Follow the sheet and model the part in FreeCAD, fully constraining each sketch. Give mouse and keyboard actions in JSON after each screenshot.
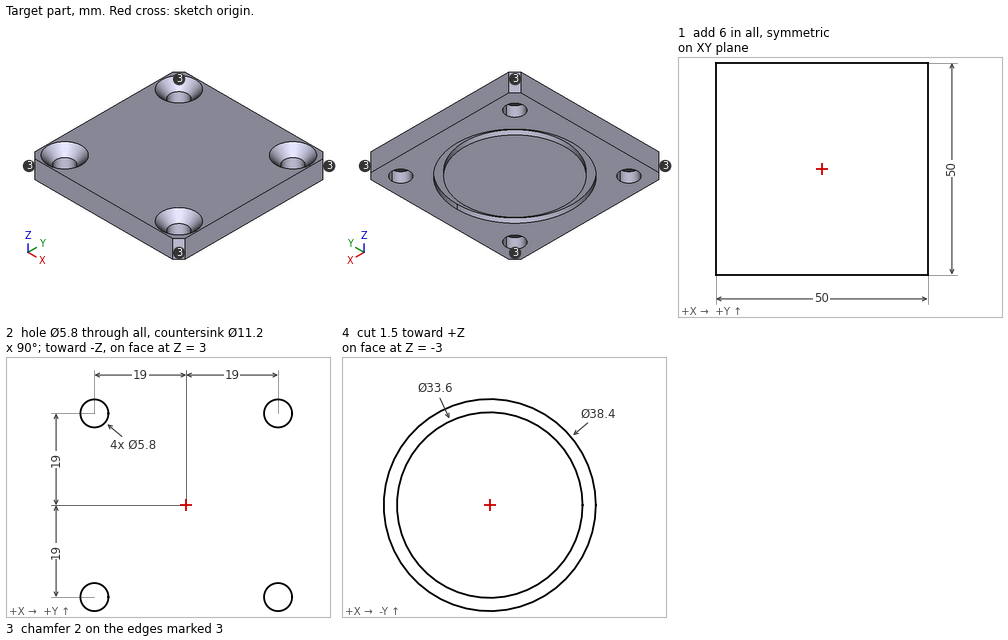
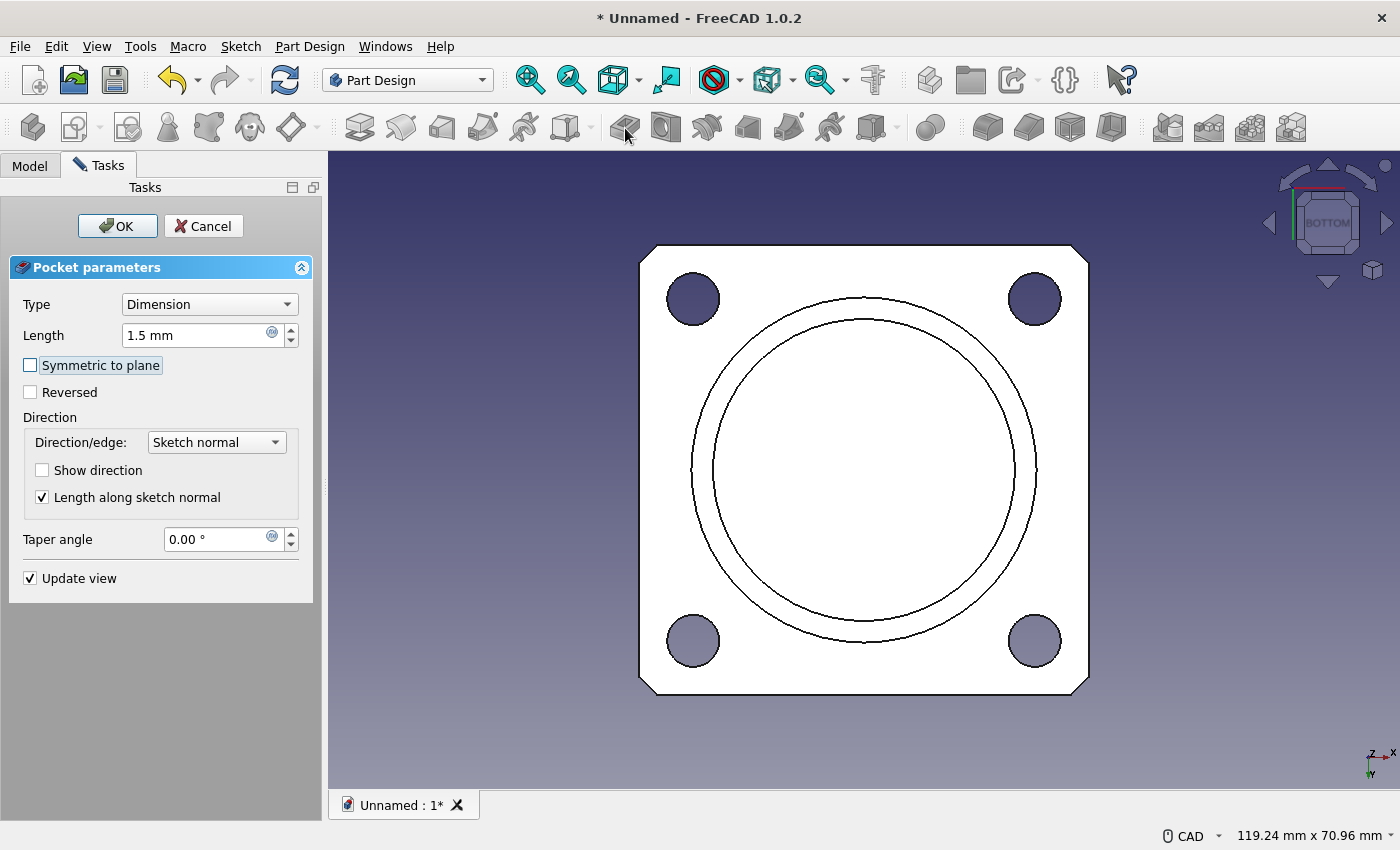
{"action": "left_click", "coordinate": [118, 226]}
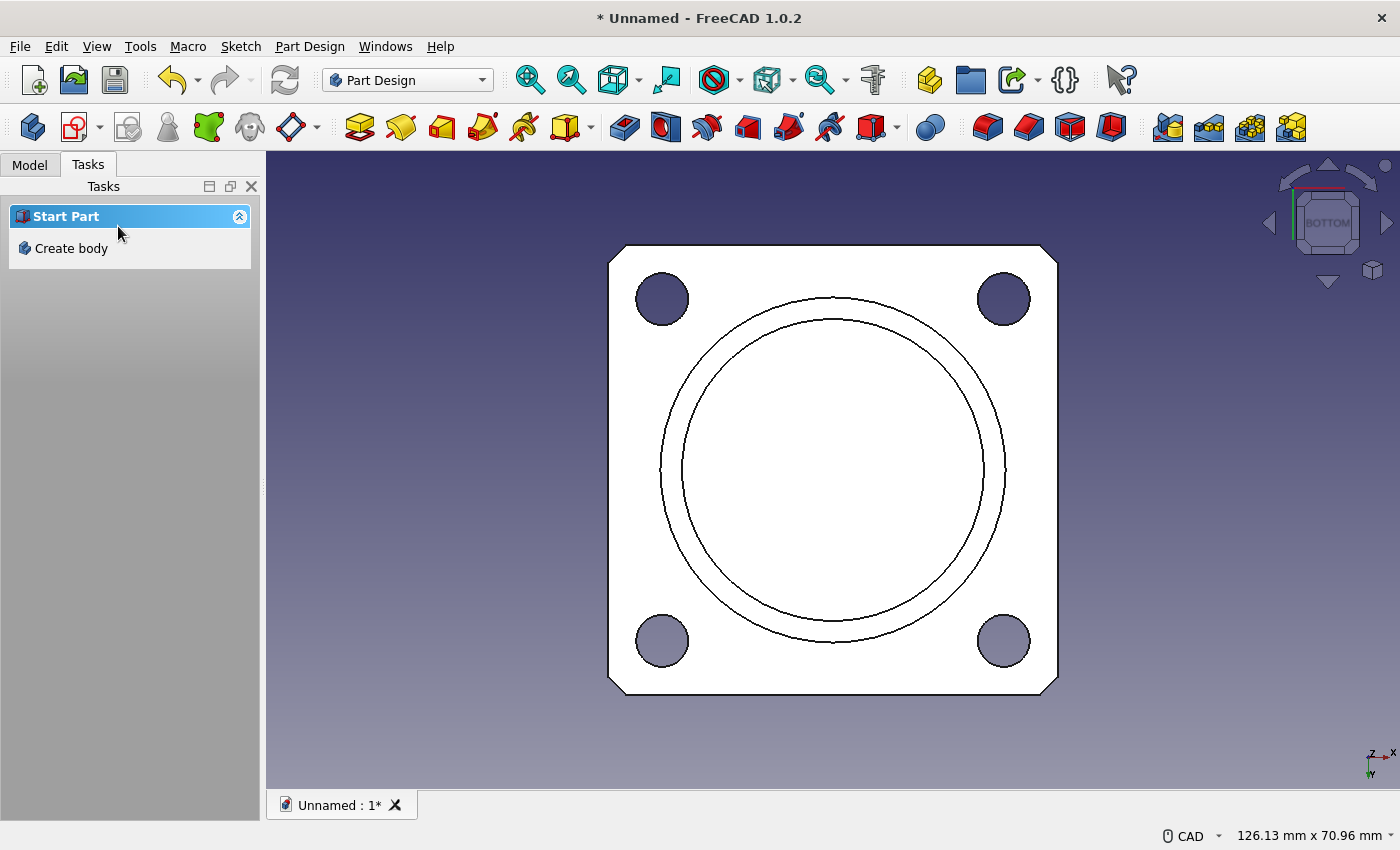
{"action": "key", "text": "0"}